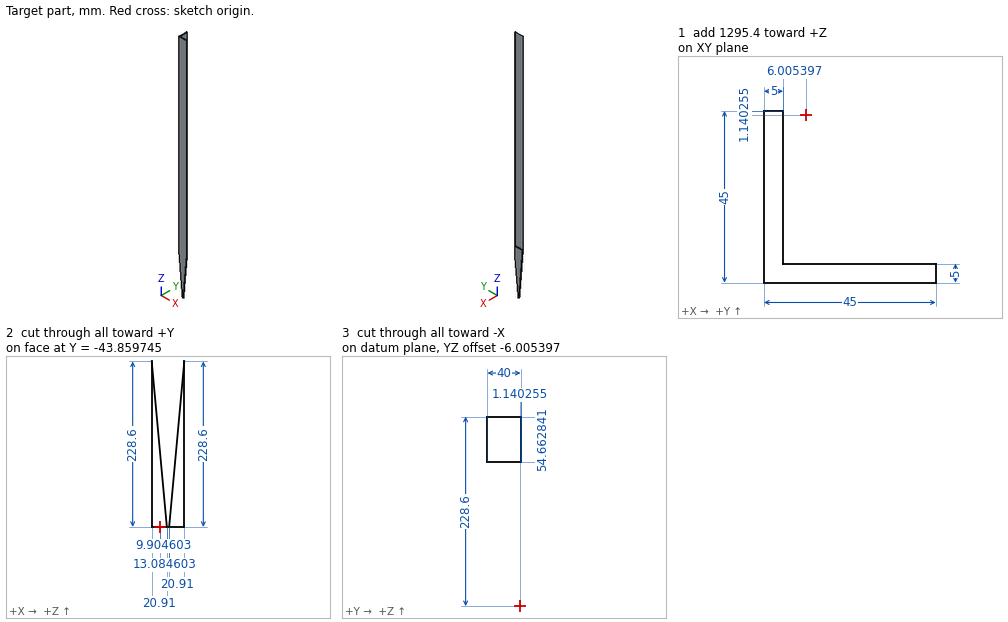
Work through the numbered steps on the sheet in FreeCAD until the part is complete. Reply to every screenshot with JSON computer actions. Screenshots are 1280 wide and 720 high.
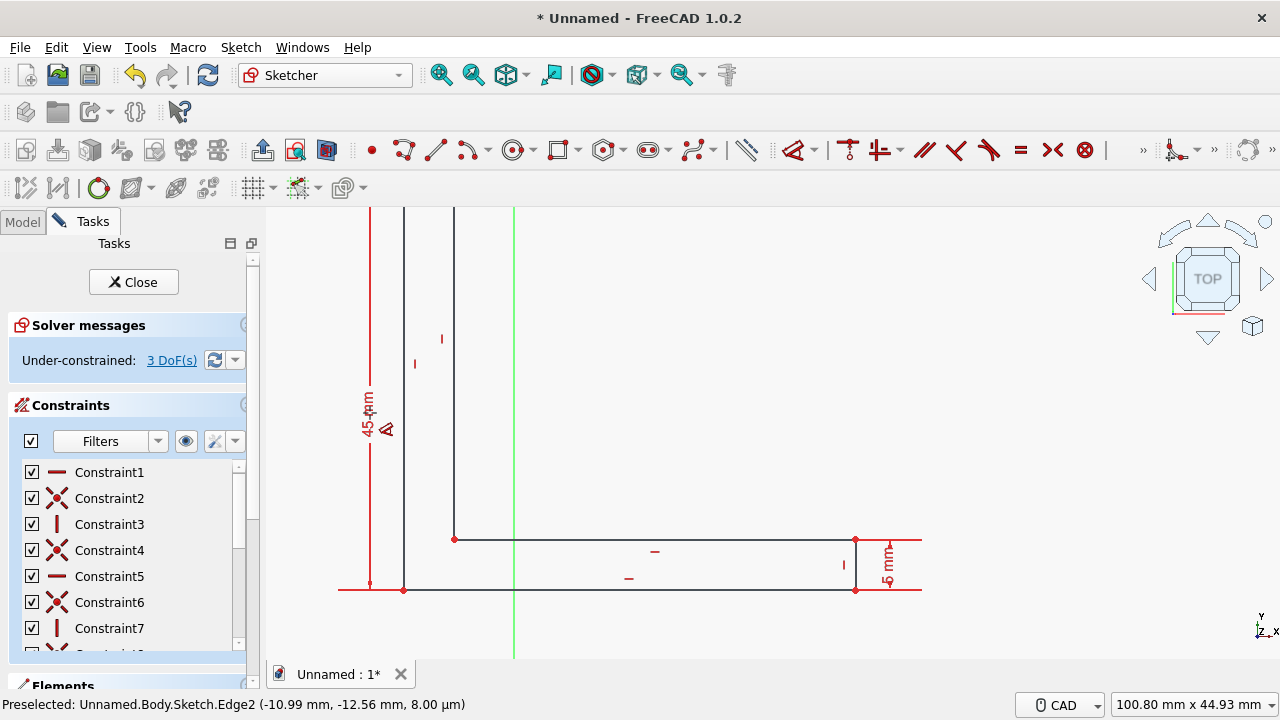
{"action": "left_click", "coordinate": [539, 590]}
{"action": "left_click", "coordinate": [630, 624]}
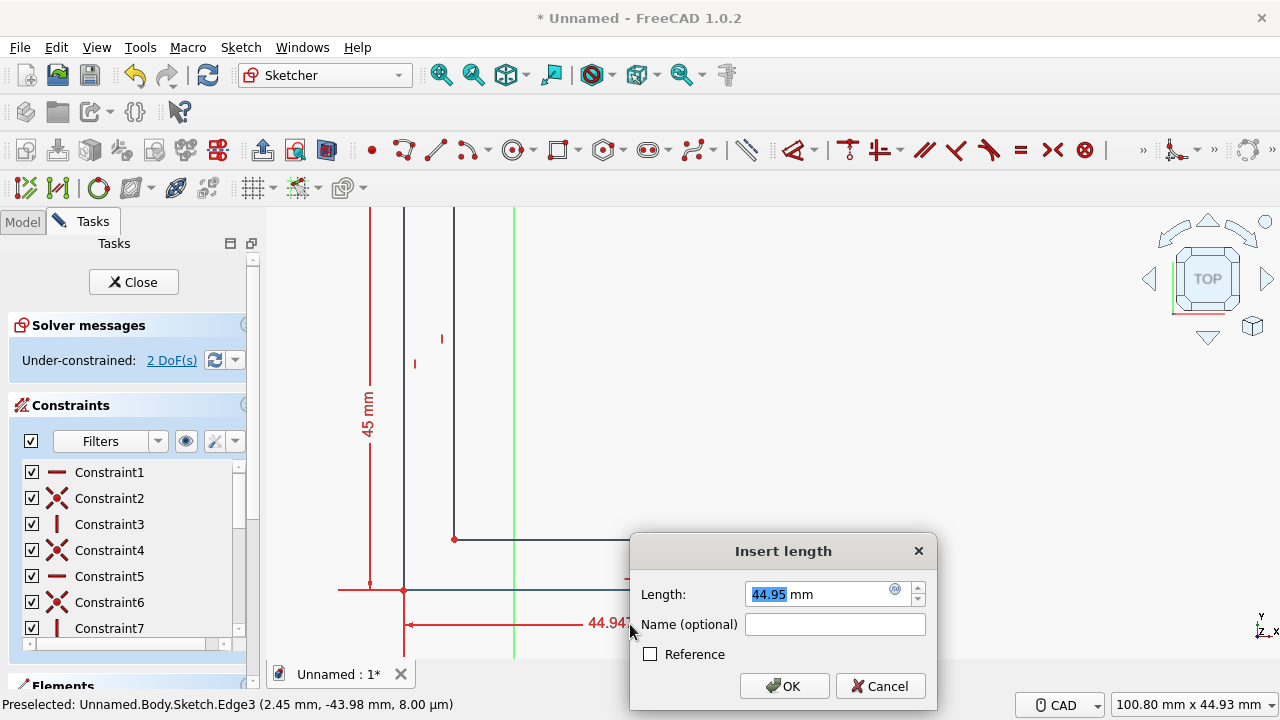
{"action": "type", "text": "45"}
{"action": "key", "text": "Return"}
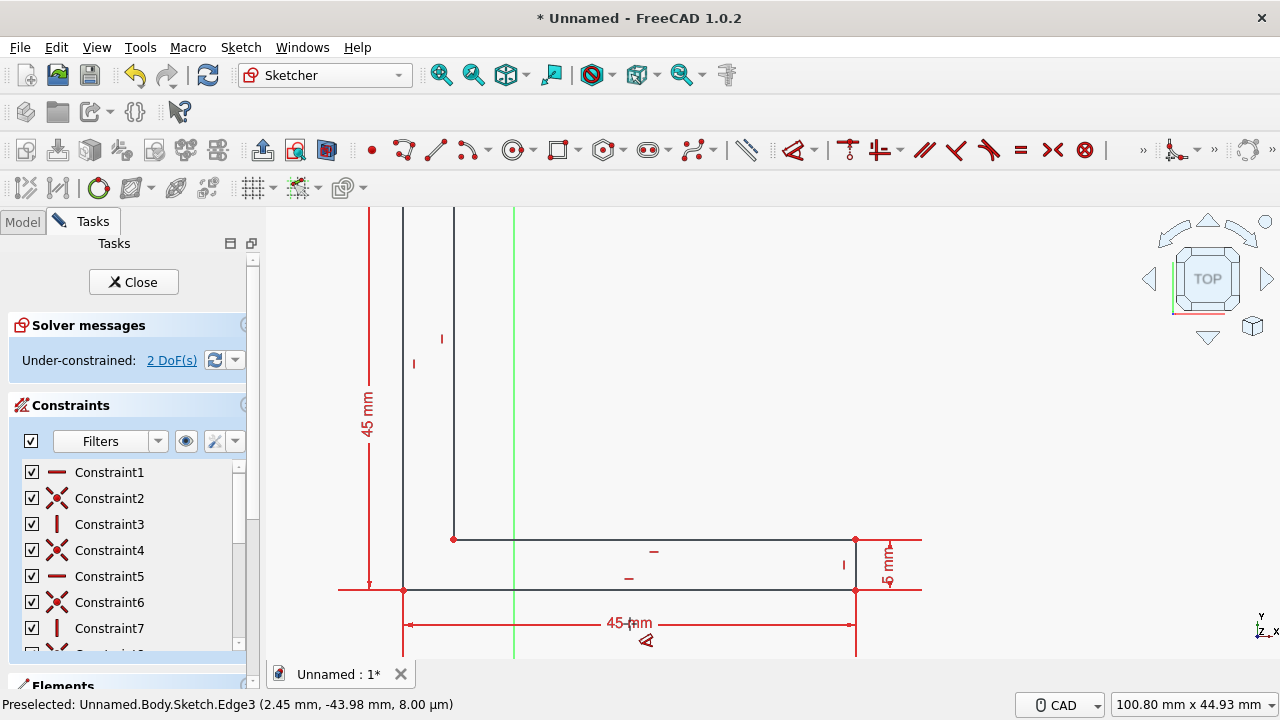
{"action": "scroll", "coordinate": [856, 576], "scroll_direction": "down", "scroll_amount": 2}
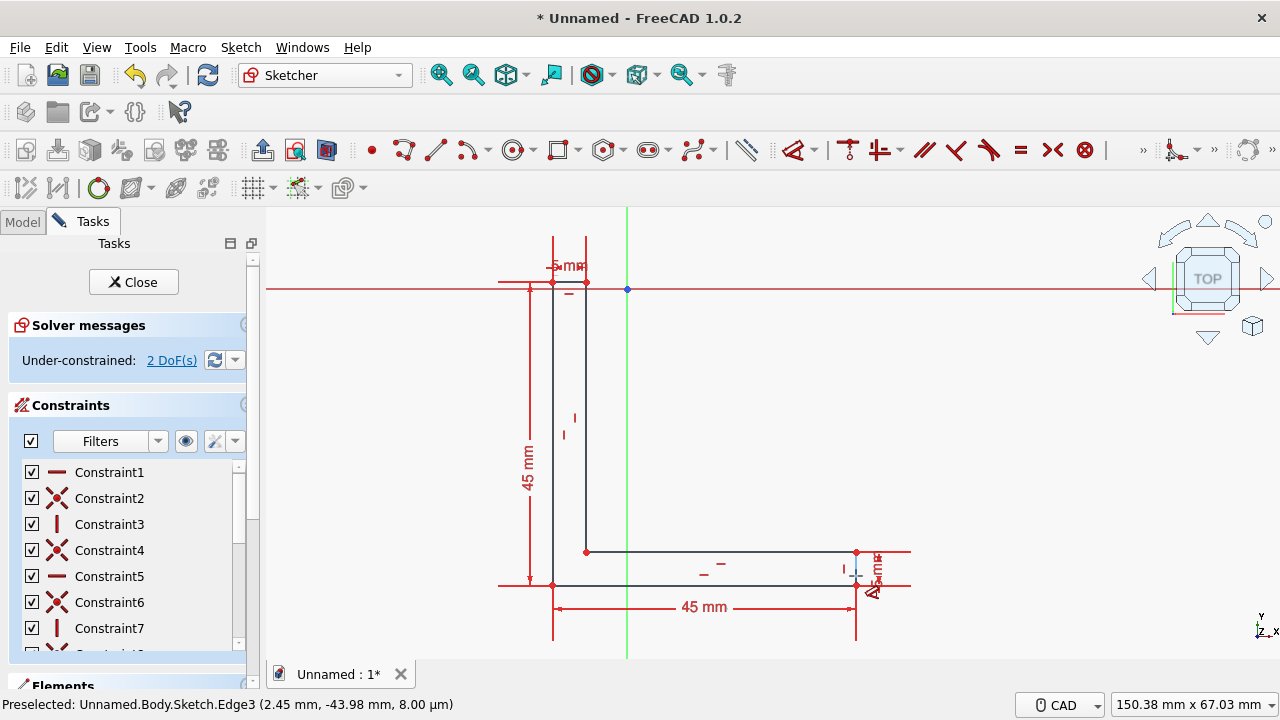
{"action": "left_click", "coordinate": [586, 282]}
{"action": "left_click", "coordinate": [607, 323]}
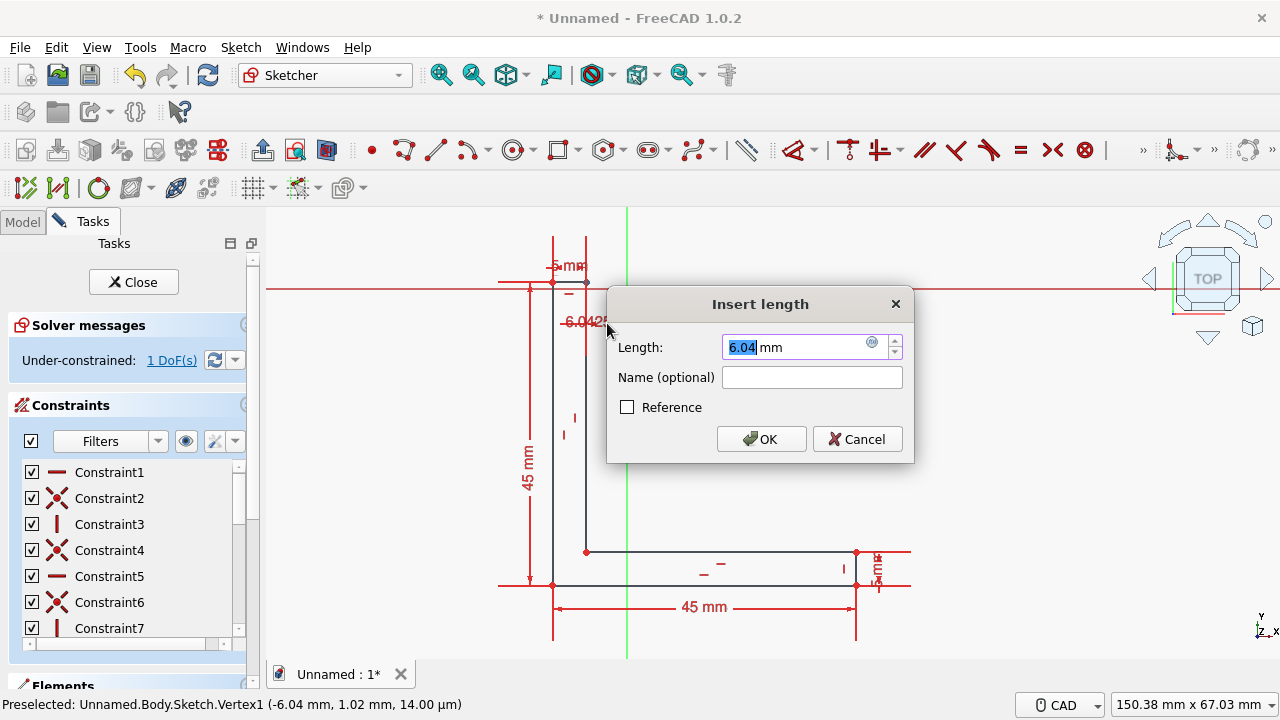
{"action": "type", "text": "6.005397"}
{"action": "key", "text": "Return"}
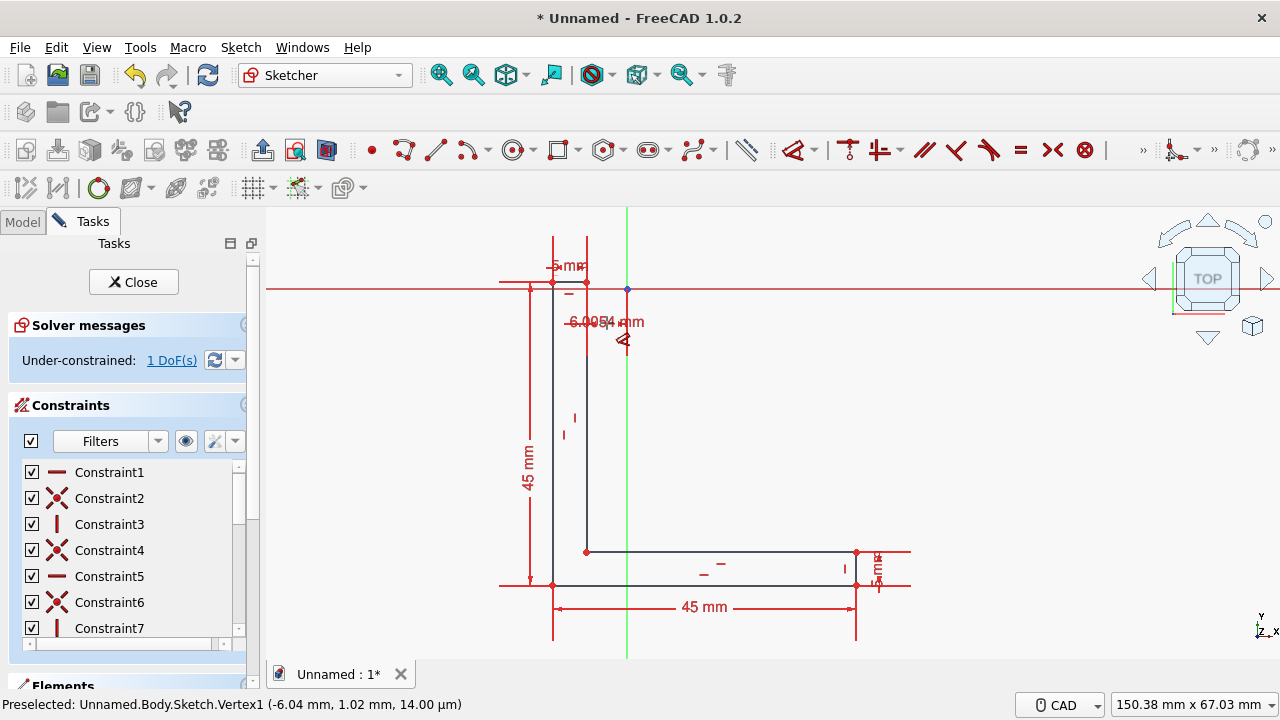
{"action": "scroll", "coordinate": [587, 282], "scroll_direction": "up", "scroll_amount": 9}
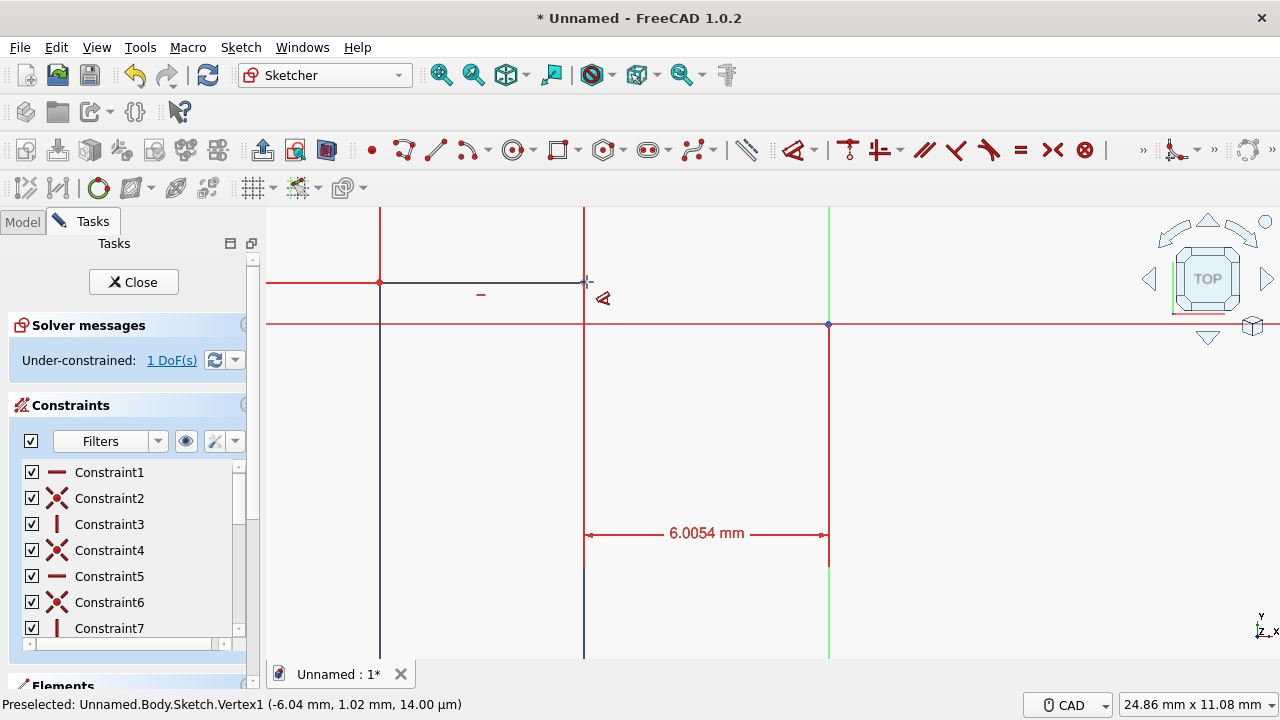
{"action": "left_click", "coordinate": [584, 283]}
{"action": "left_click", "coordinate": [550, 304]}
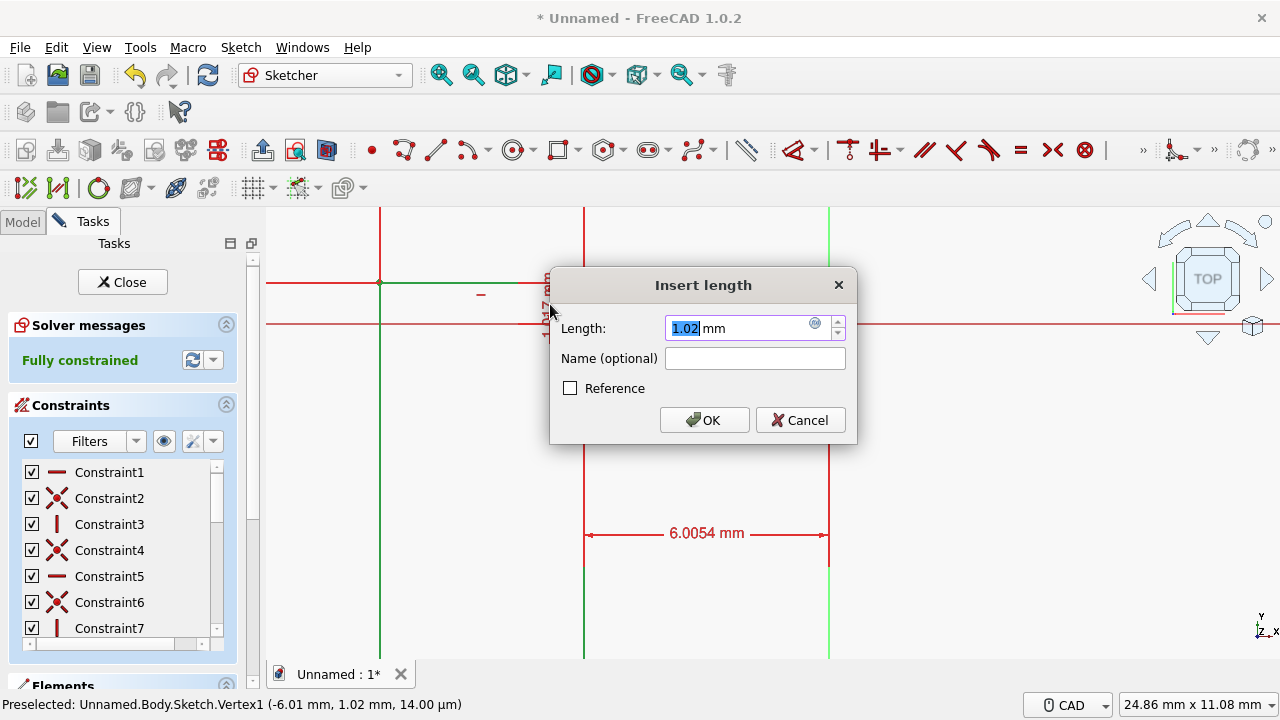
{"action": "type", "text": "1.140255"}
{"action": "key", "text": "Return"}
{"action": "key", "text": "Escape"}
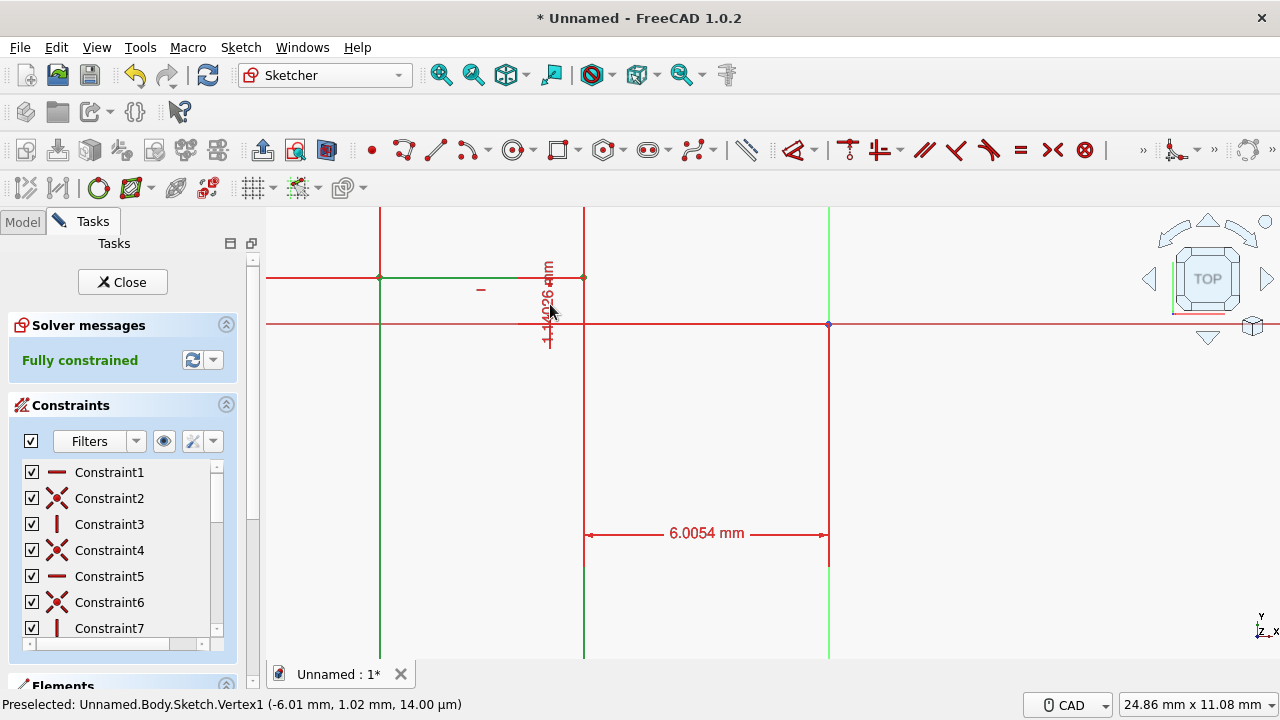
{"action": "left_click", "coordinate": [123, 282]}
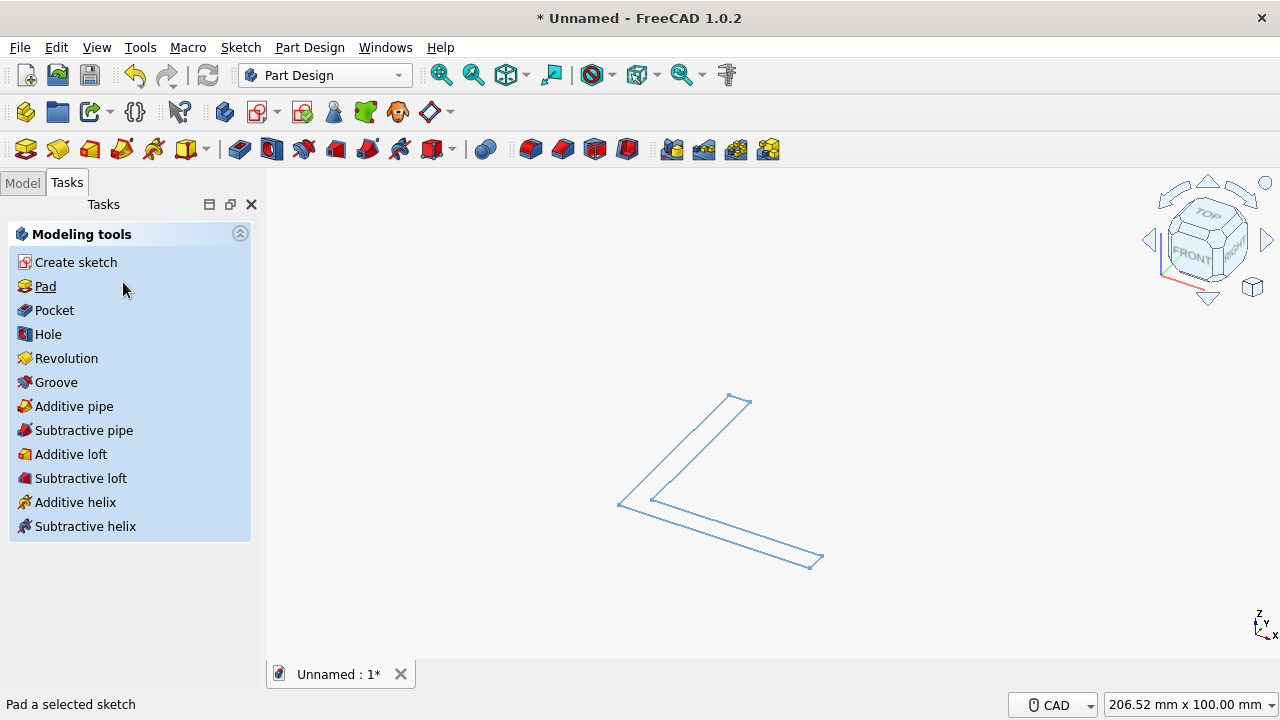
{"action": "left_click", "coordinate": [26, 150]}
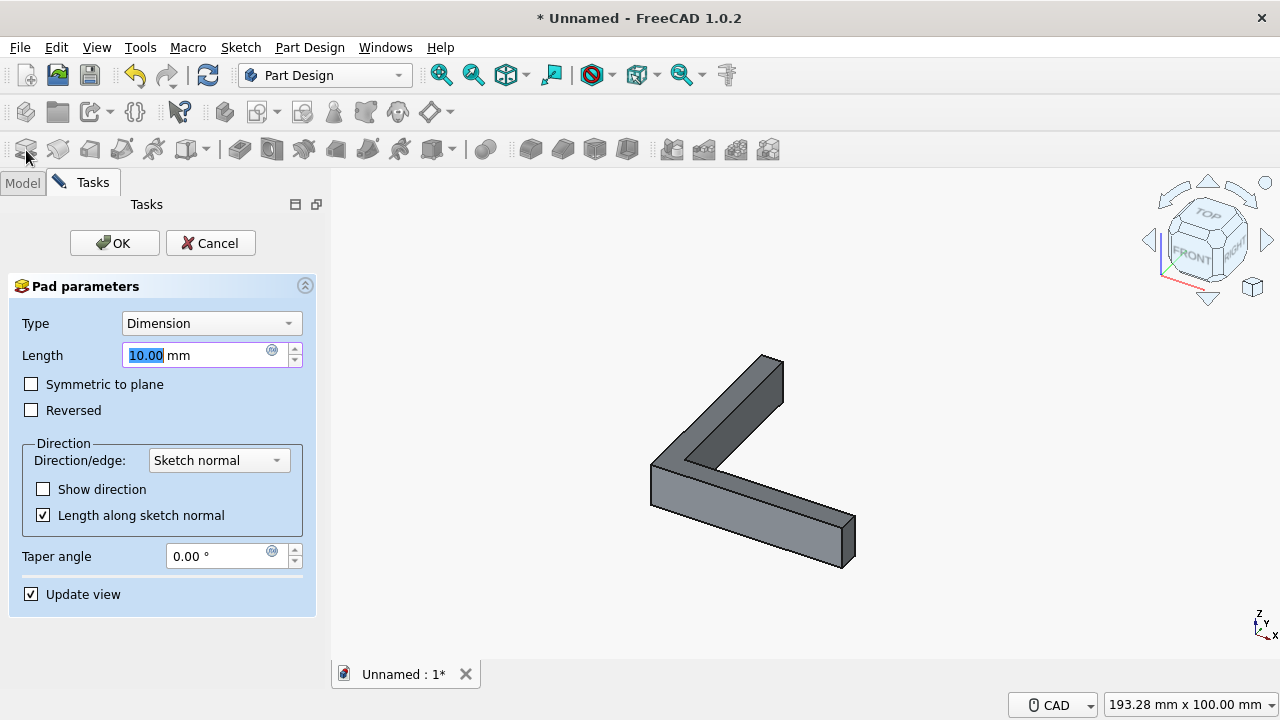
{"action": "type", "text": "1295.4"}
{"action": "key", "text": "Tab"}